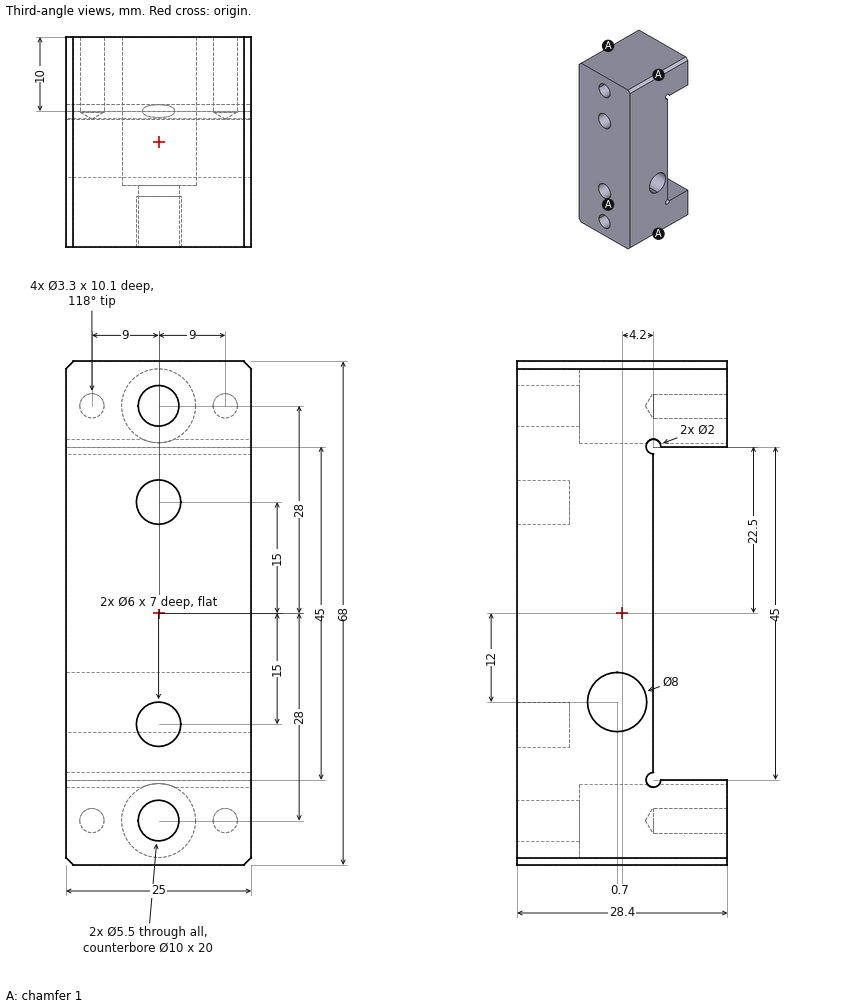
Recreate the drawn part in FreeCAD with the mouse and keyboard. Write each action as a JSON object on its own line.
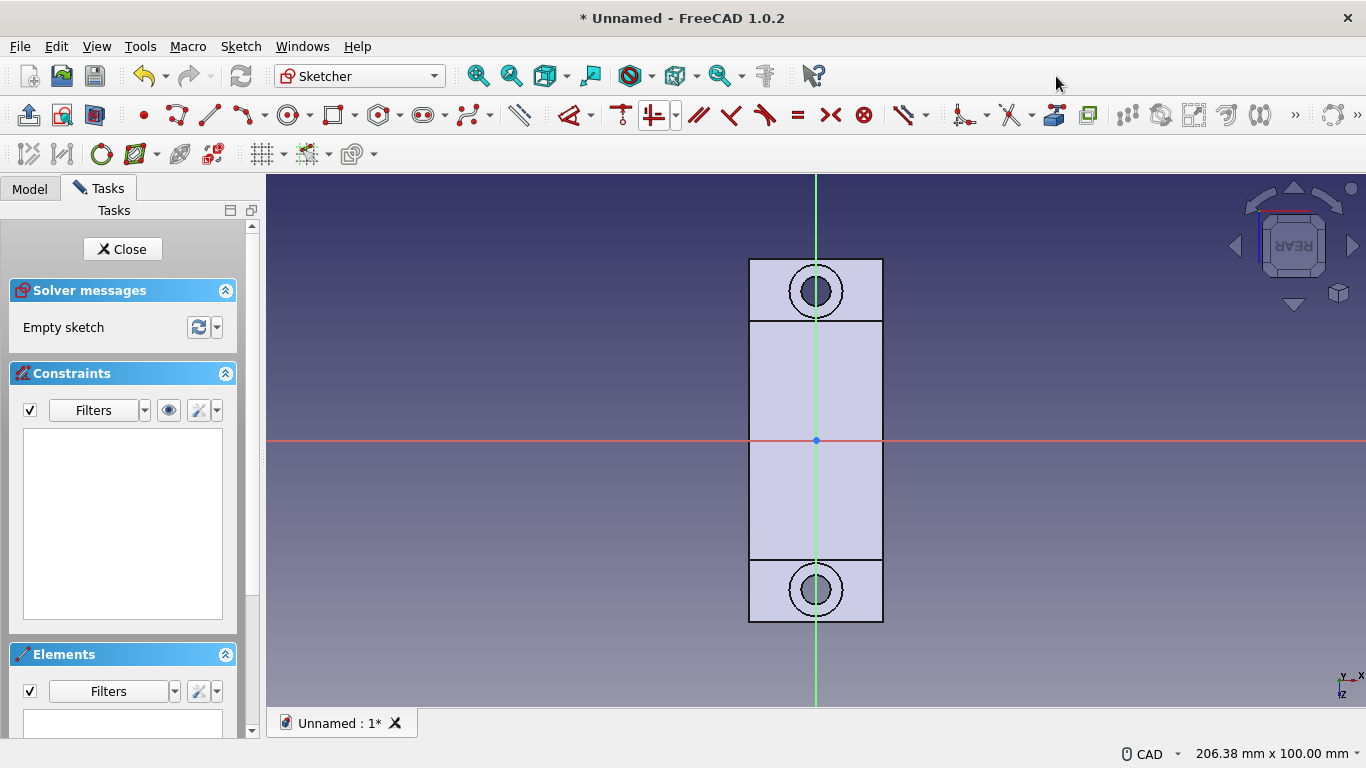
{"action": "left_click", "coordinate": [288, 116]}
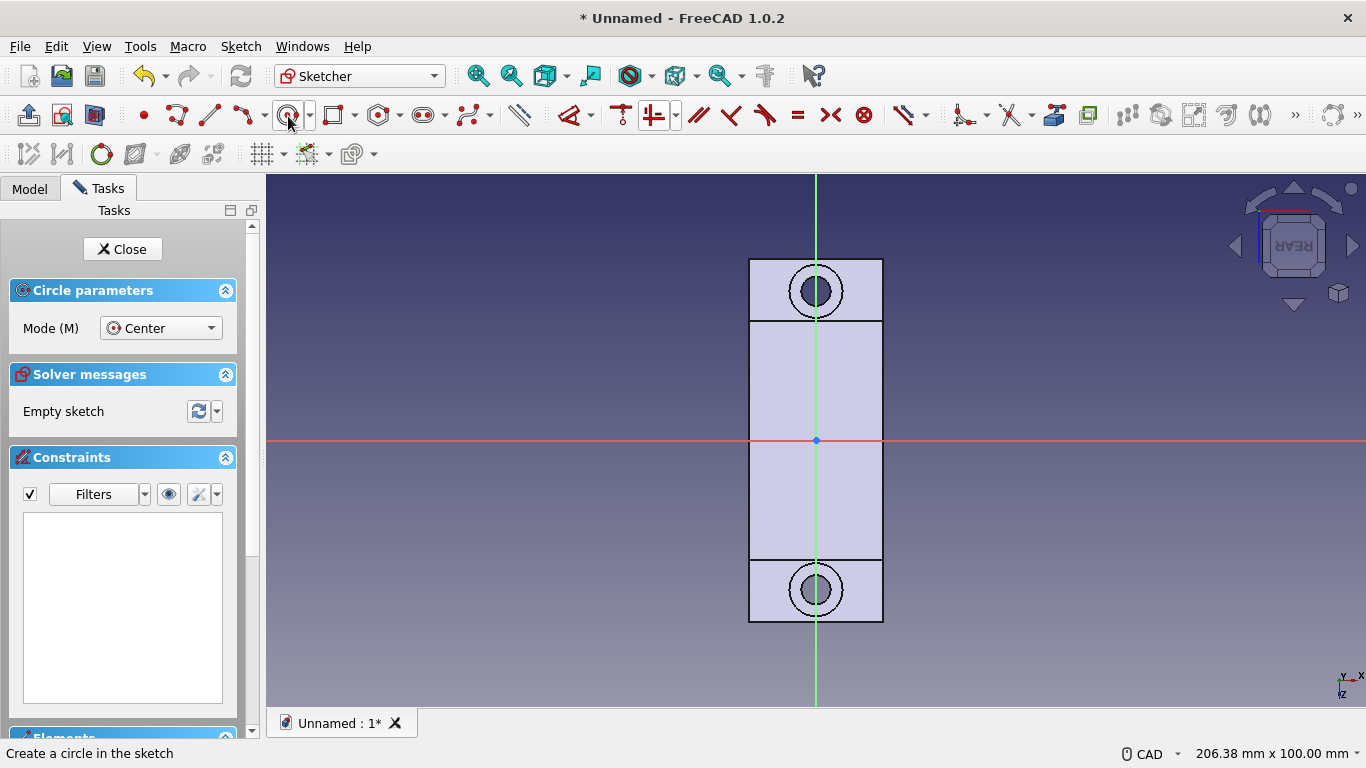
{"action": "scroll", "coordinate": [768, 590], "scroll_direction": "up", "scroll_amount": 5}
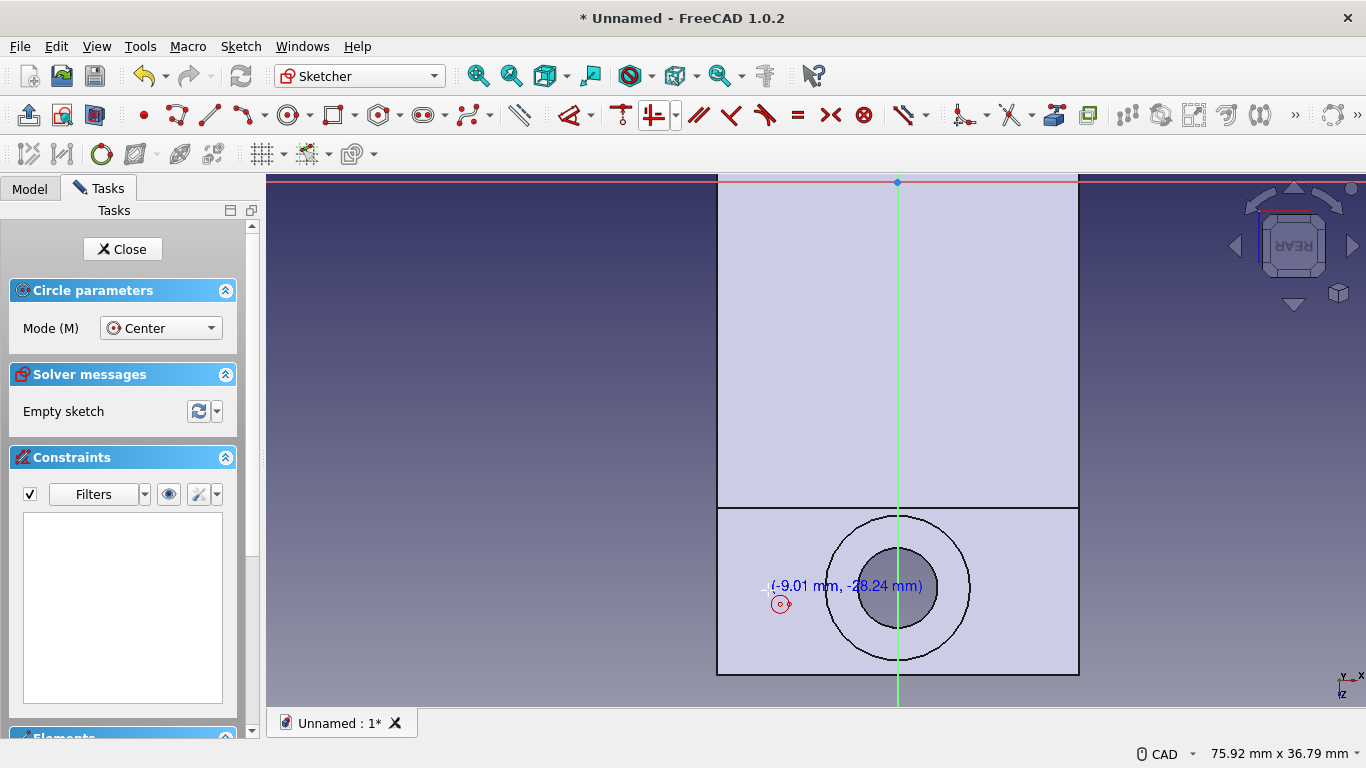
{"action": "left_click", "coordinate": [767, 588]}
{"action": "left_click", "coordinate": [784, 571]}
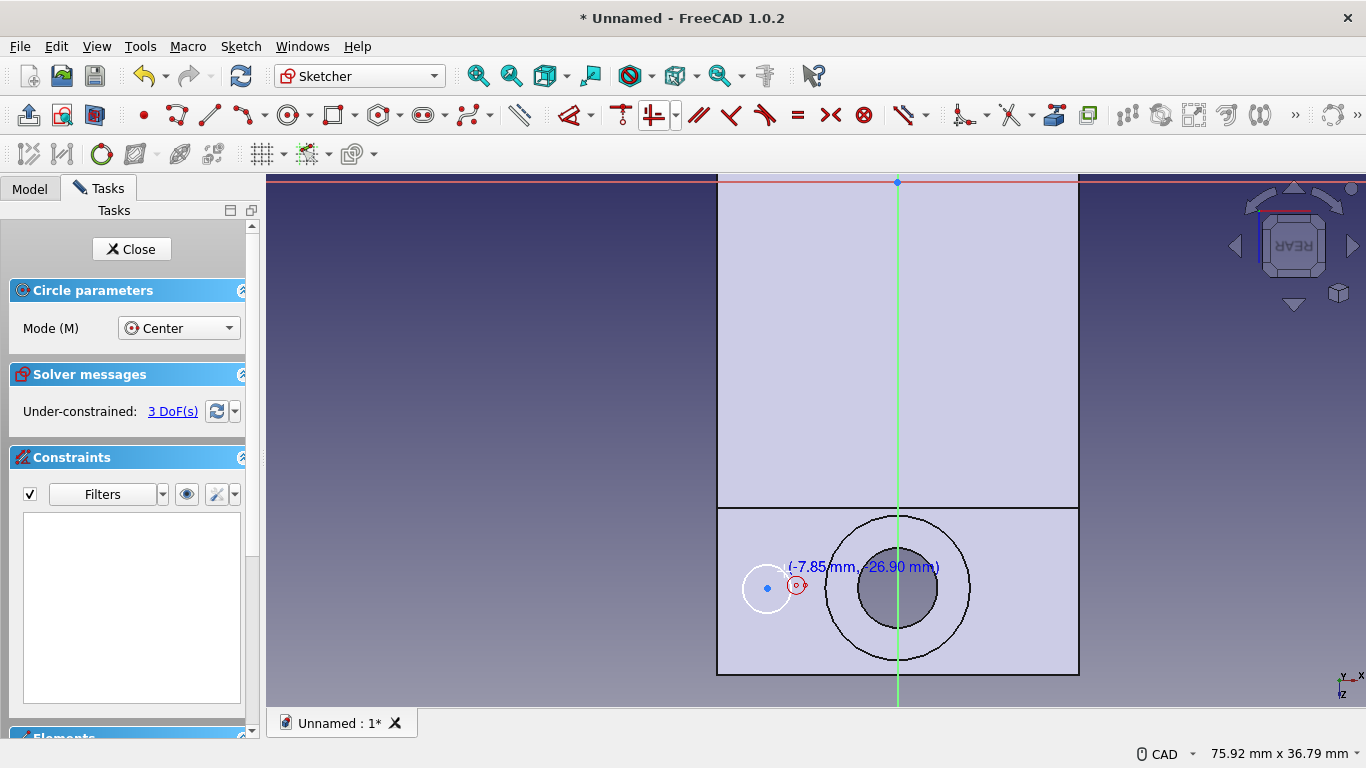
{"action": "left_click", "coordinate": [1028, 588]}
{"action": "left_click", "coordinate": [1045, 571]}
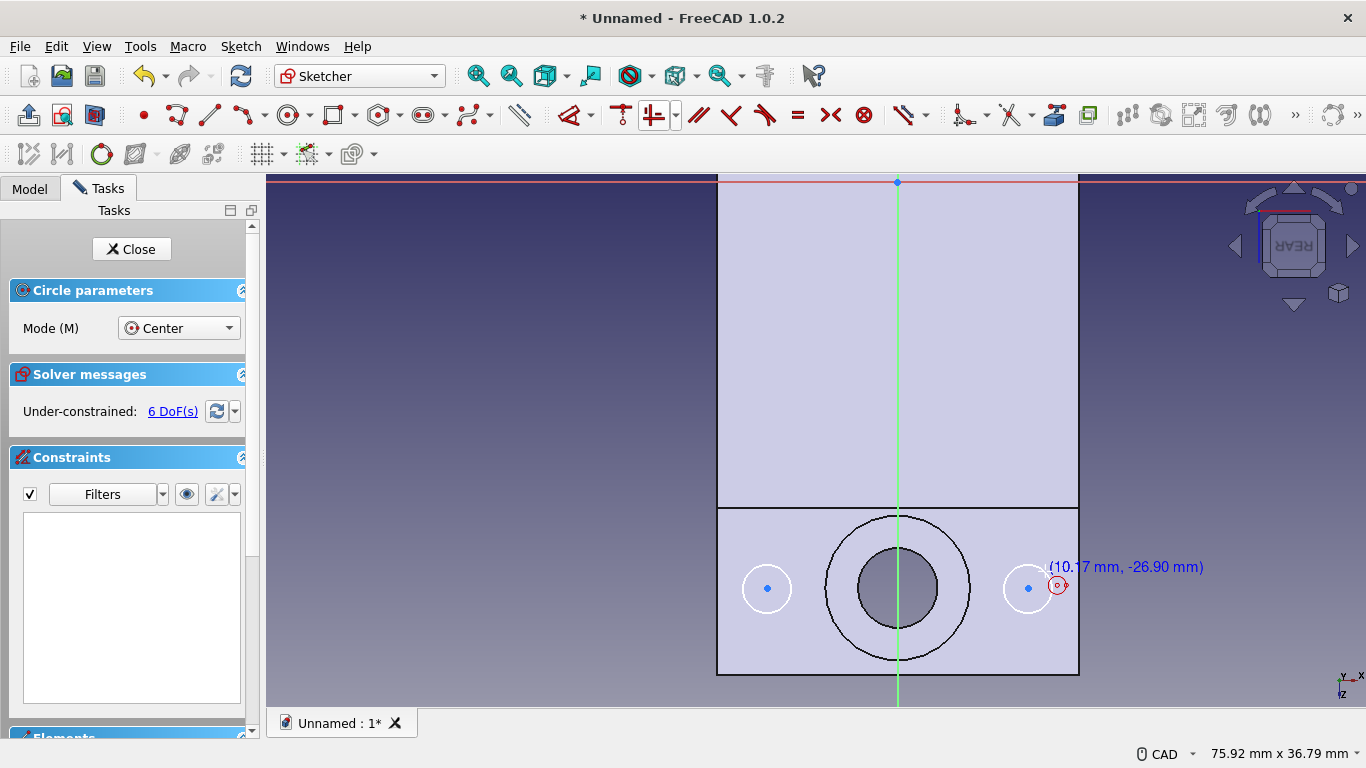
{"action": "scroll", "coordinate": [660, 591], "scroll_direction": "down", "scroll_amount": 5}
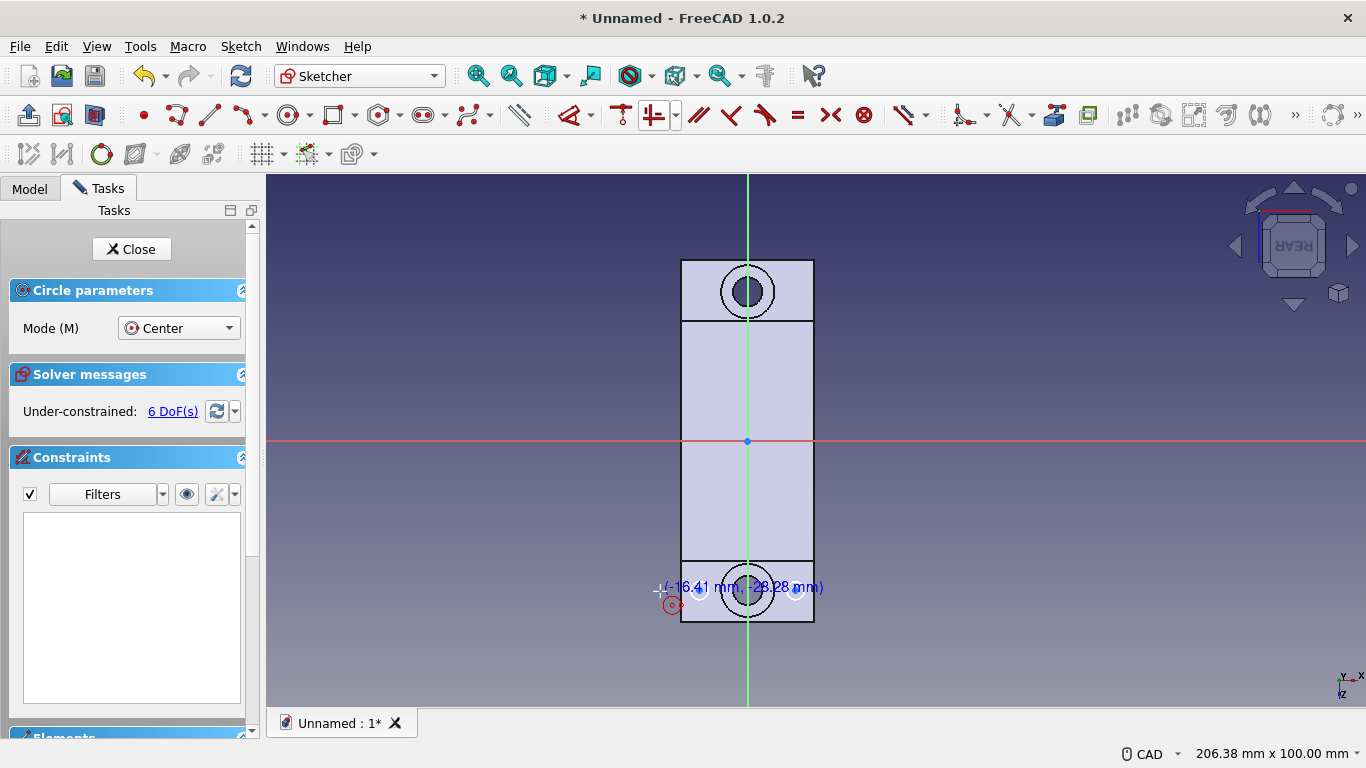
{"action": "scroll", "coordinate": [796, 292], "scroll_direction": "up", "scroll_amount": 5}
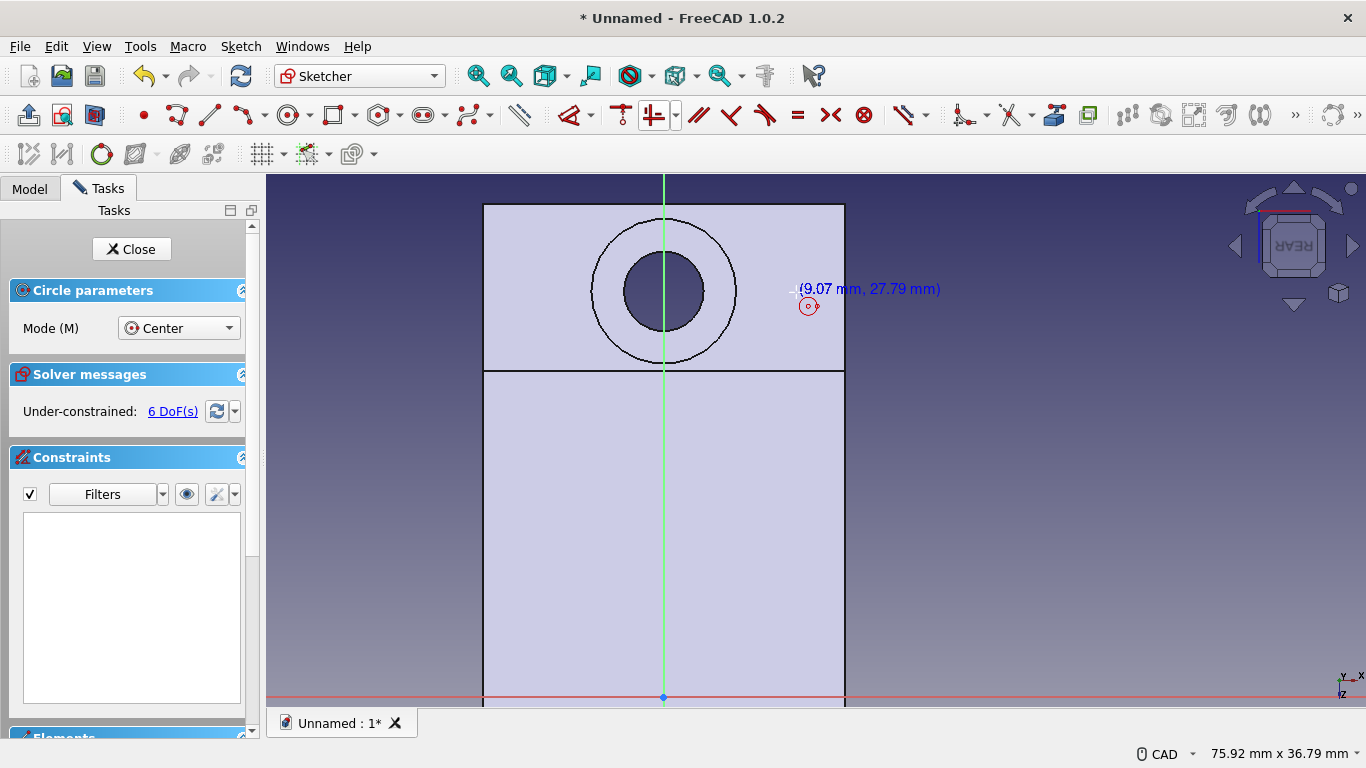
{"action": "left_click", "coordinate": [794, 291]}
{"action": "left_click", "coordinate": [811, 274]}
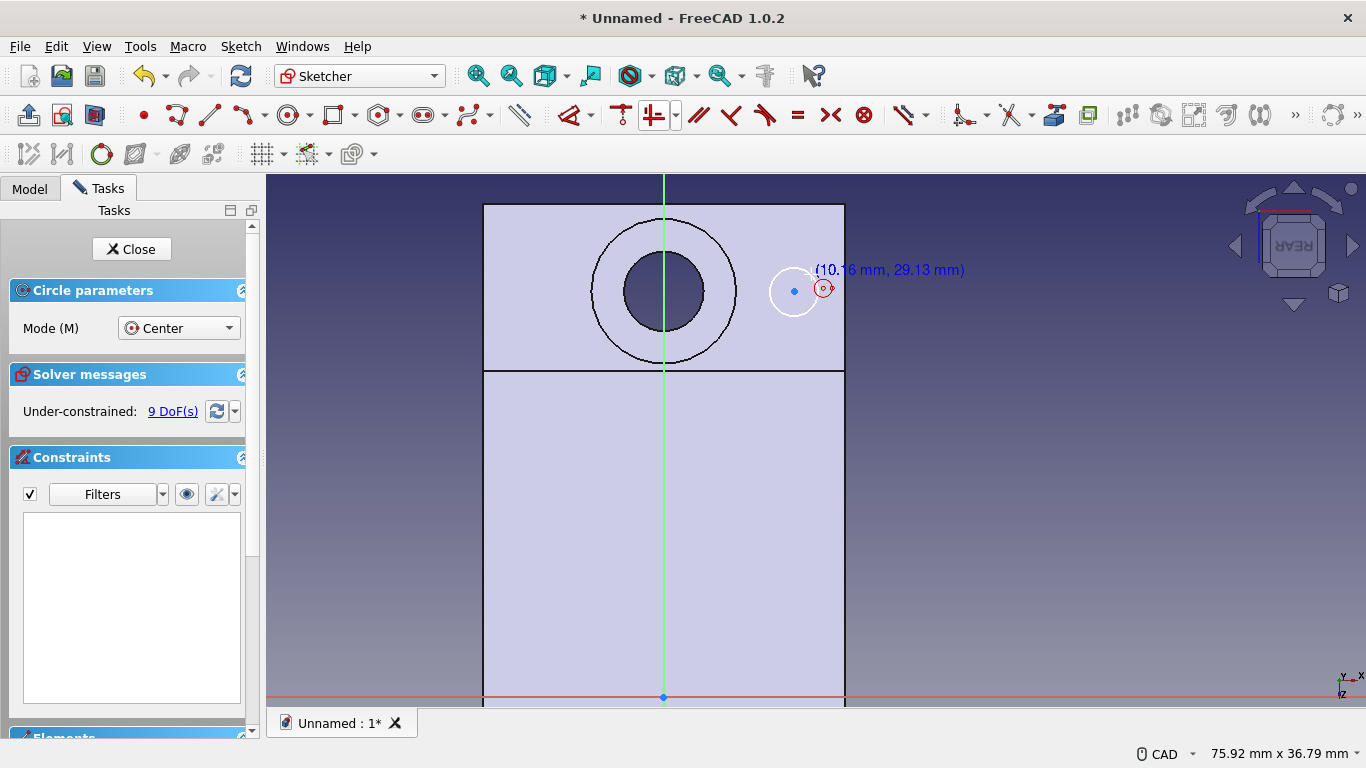
{"action": "left_click", "coordinate": [533, 291]}
{"action": "left_click", "coordinate": [550, 274]}
{"action": "key", "text": "Escape"}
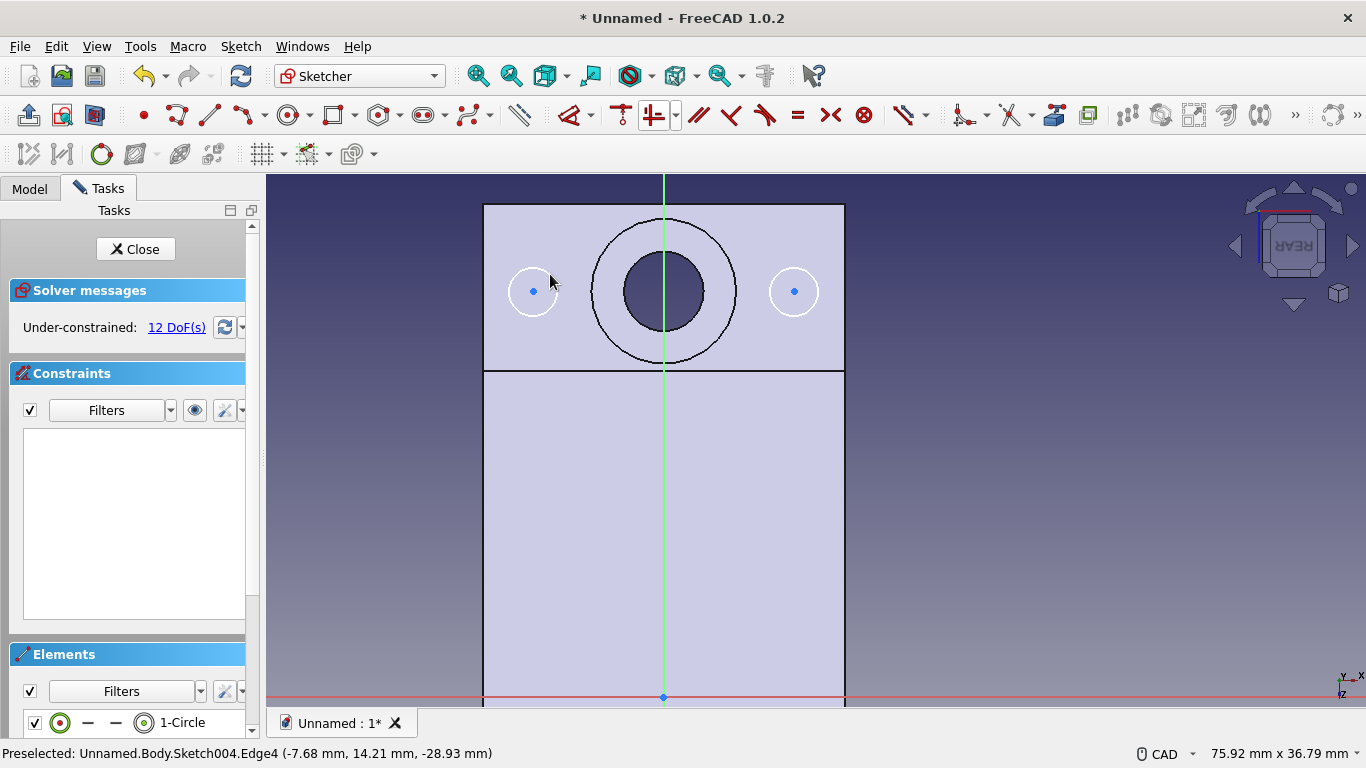
{"action": "scroll", "coordinate": [796, 291], "scroll_direction": "down", "scroll_amount": 5}